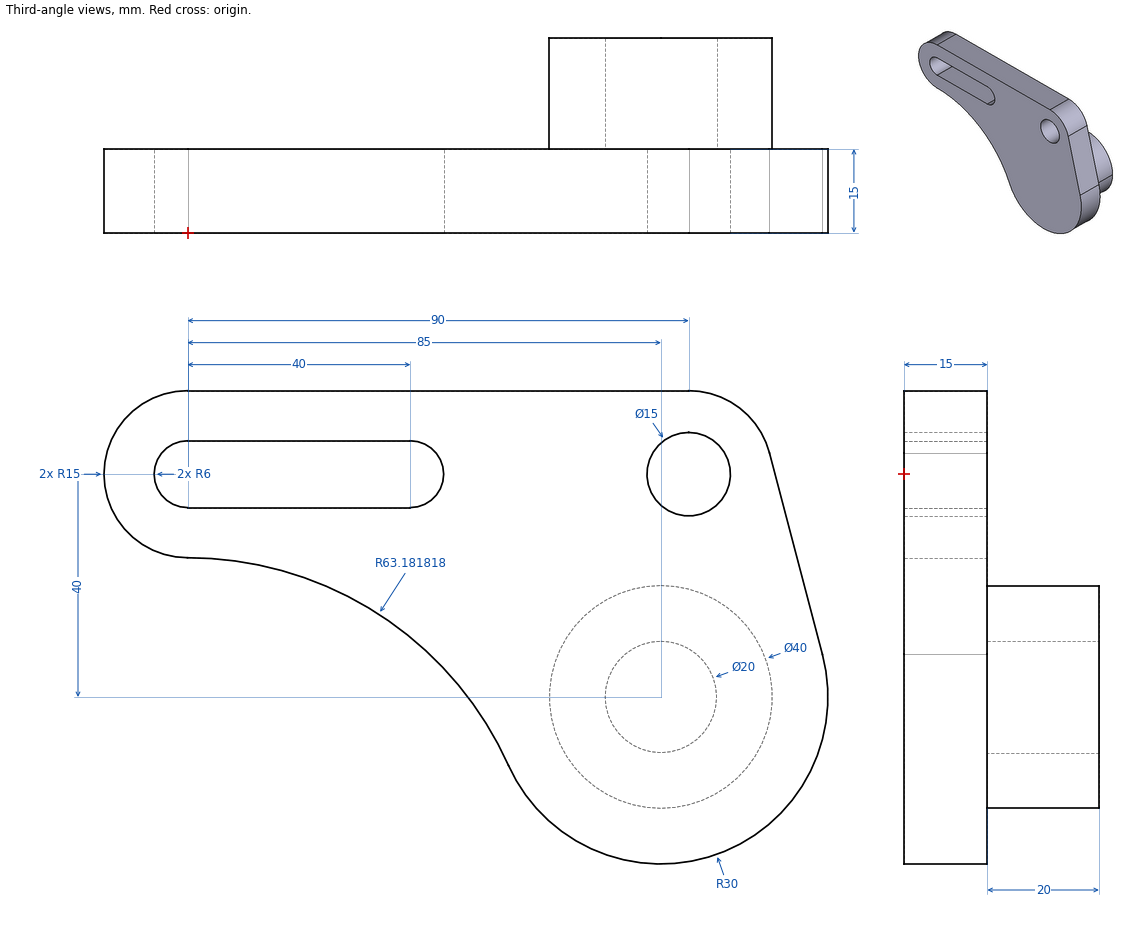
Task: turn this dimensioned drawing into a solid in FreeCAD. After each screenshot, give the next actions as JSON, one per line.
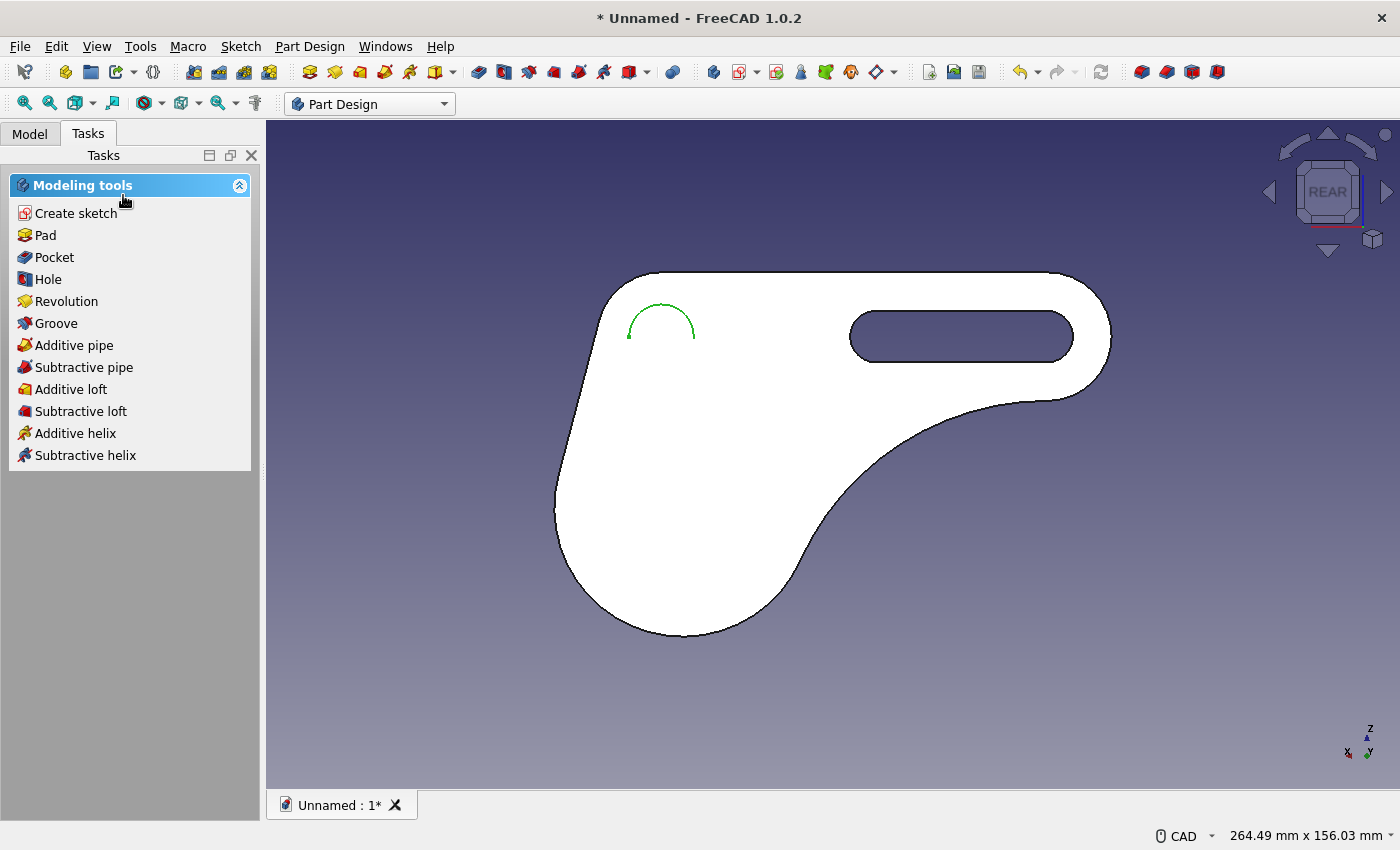
{"action": "left_click", "coordinate": [479, 72]}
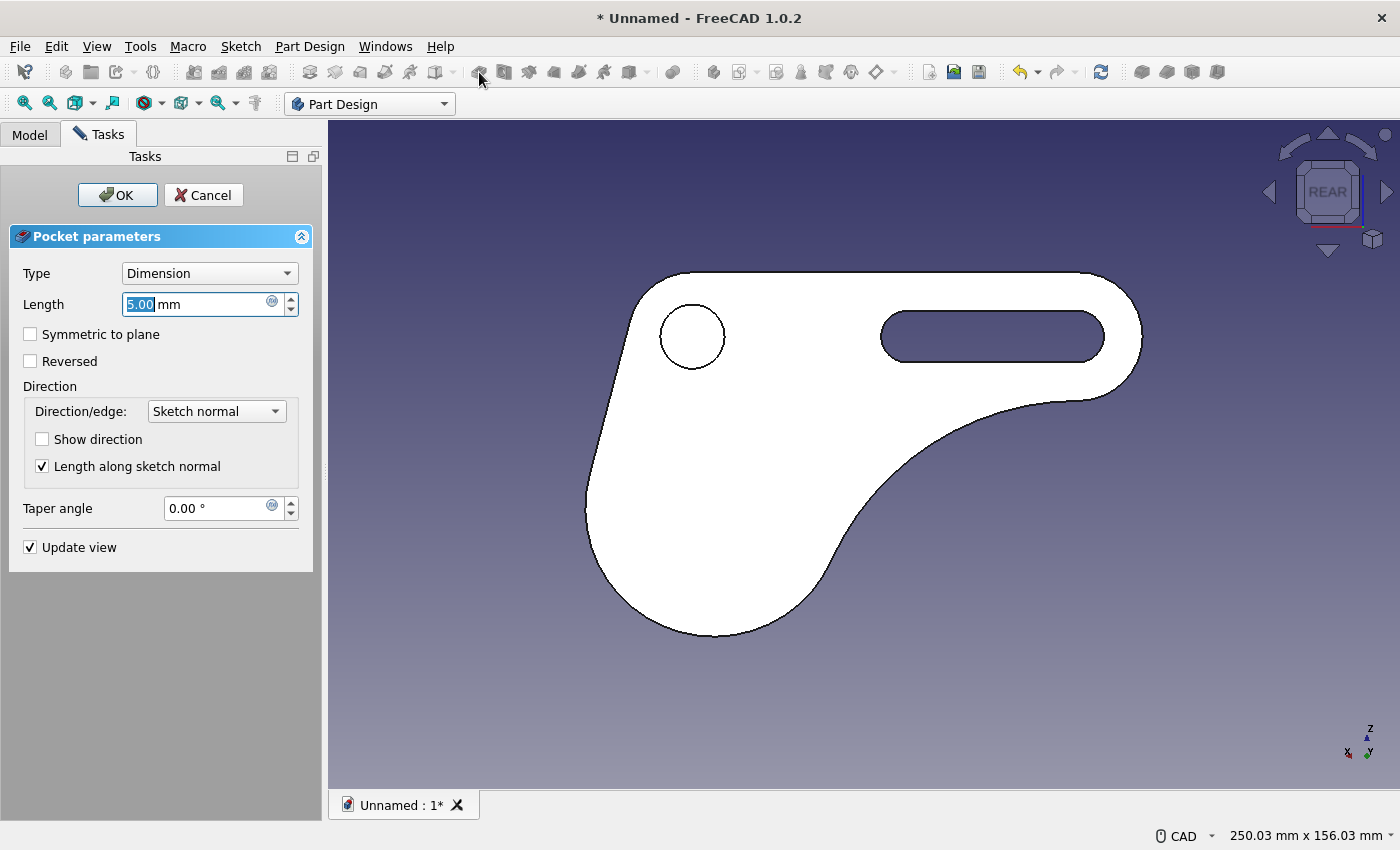
{"action": "type", "text": "15"}
{"action": "key", "text": "Tab"}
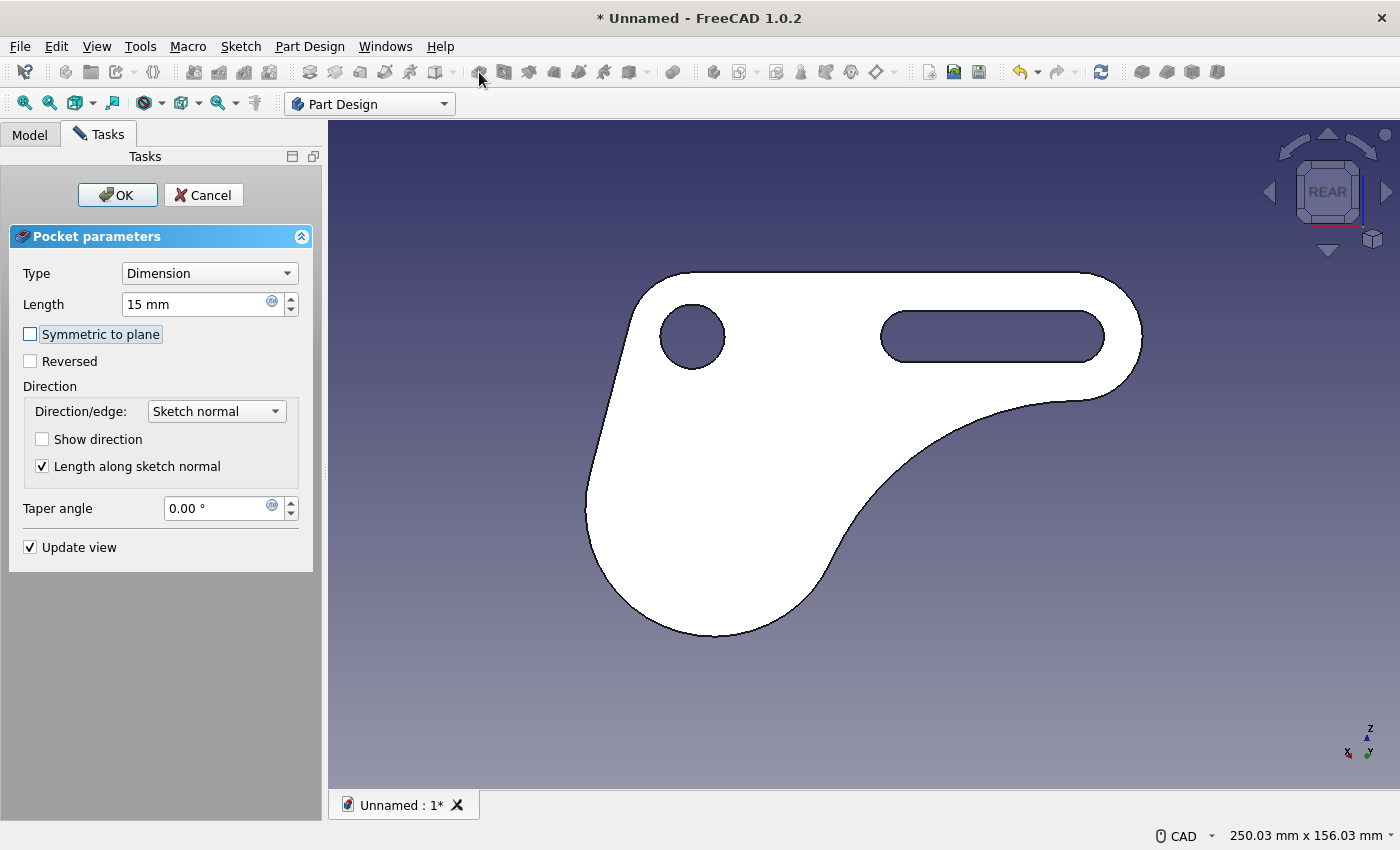
{"action": "left_click", "coordinate": [118, 195]}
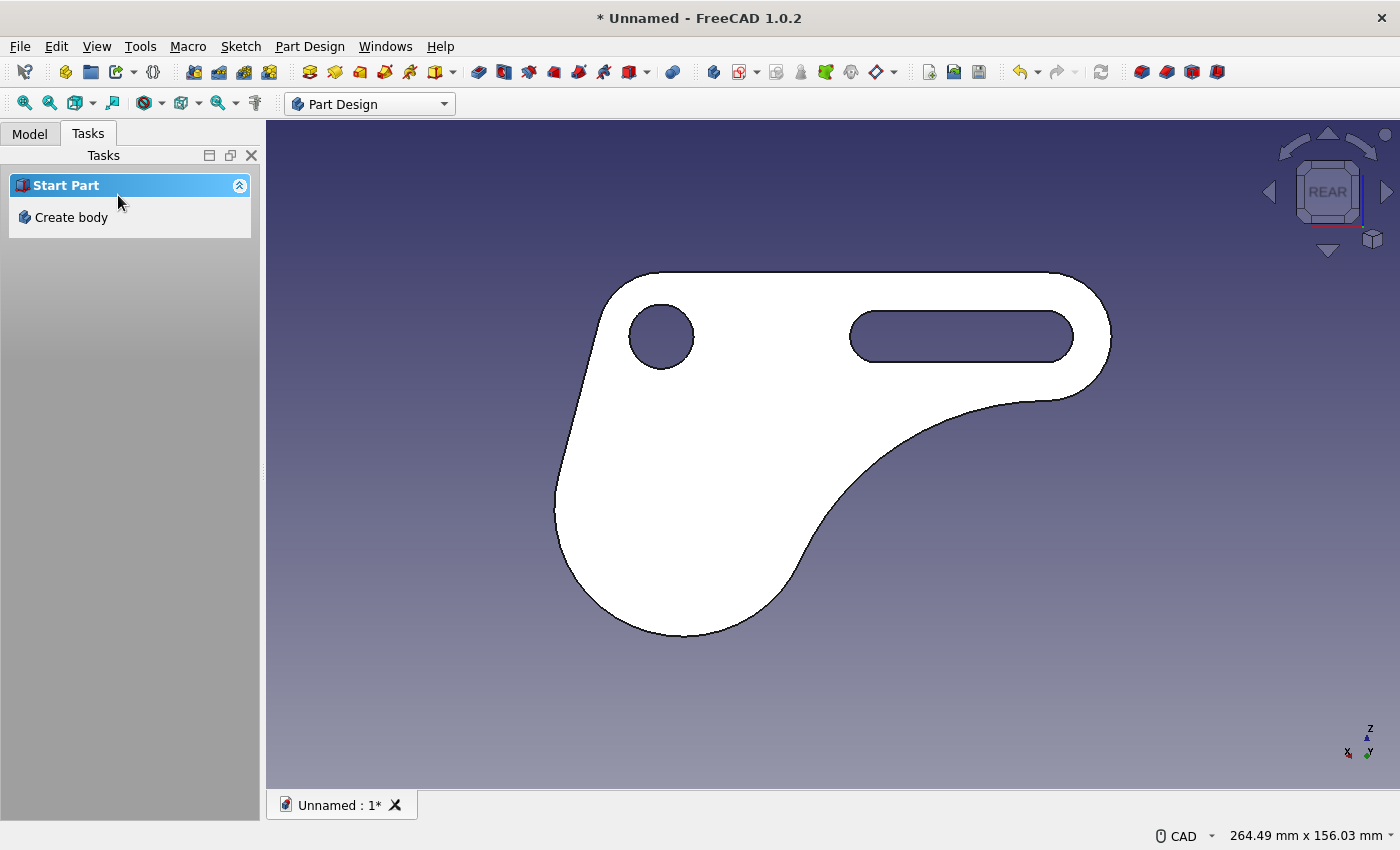
{"action": "left_click", "coordinate": [674, 506]}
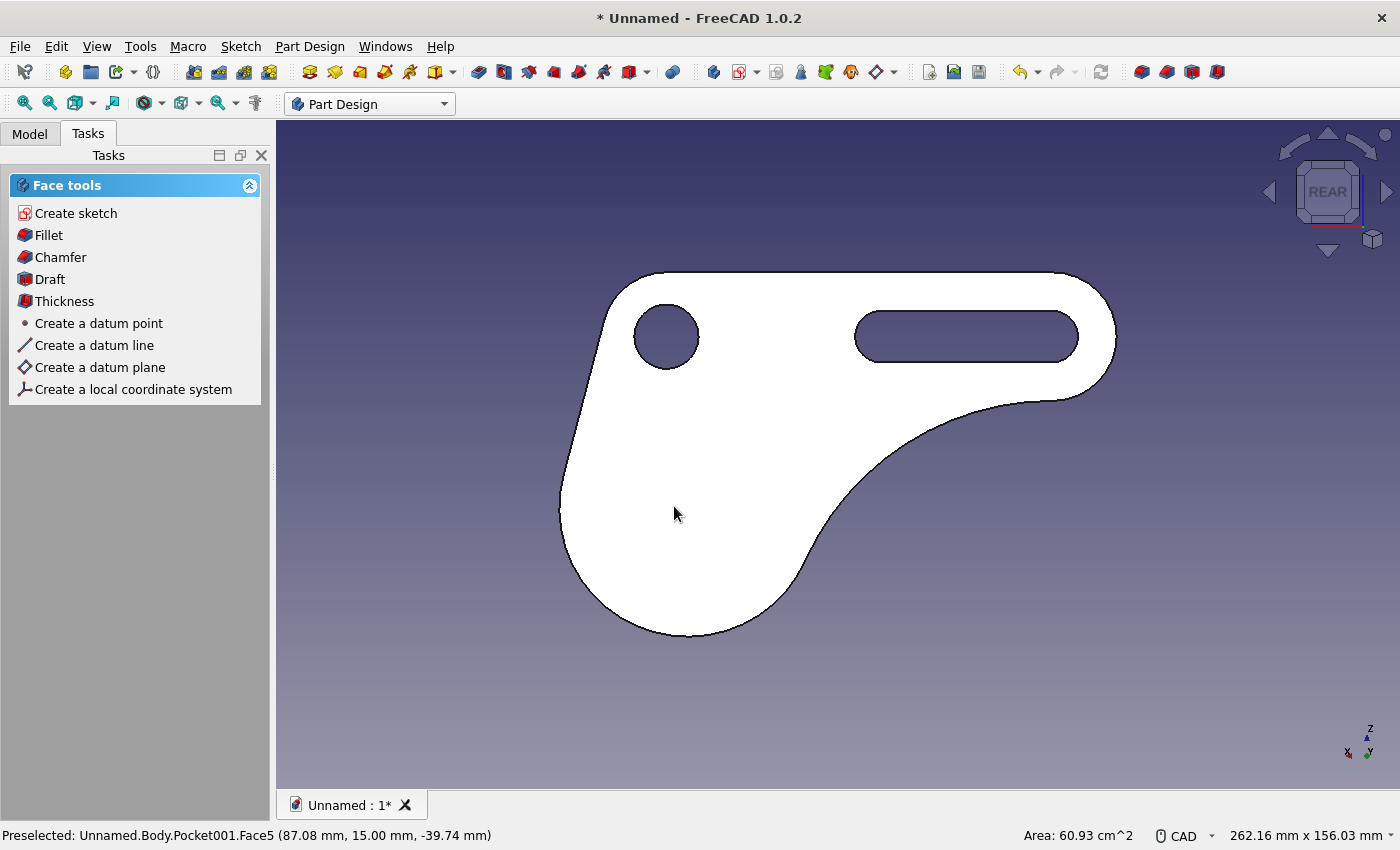
{"action": "left_click", "coordinate": [738, 72]}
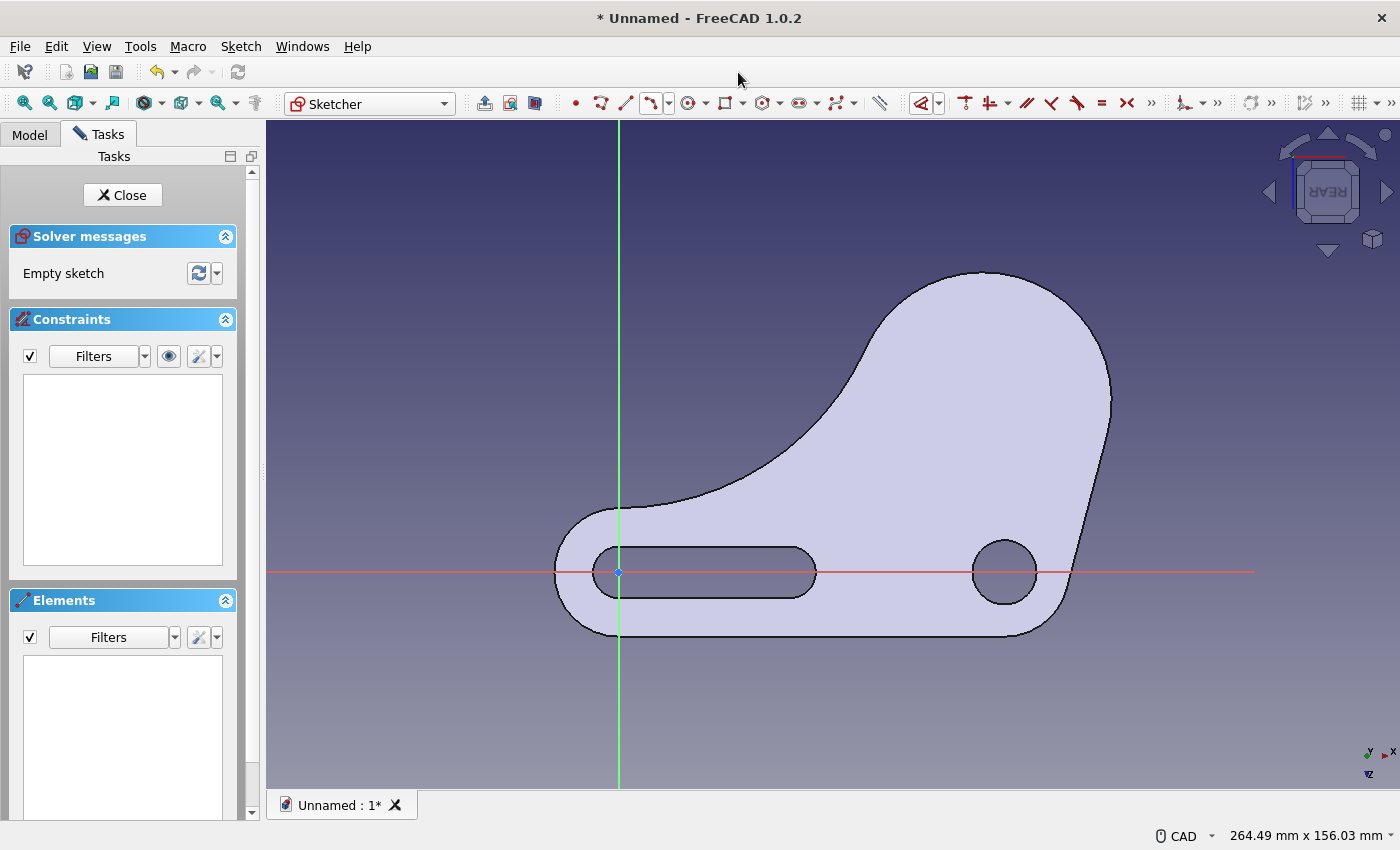
{"action": "scroll", "coordinate": [1110, 370], "scroll_direction": "up", "scroll_amount": 5}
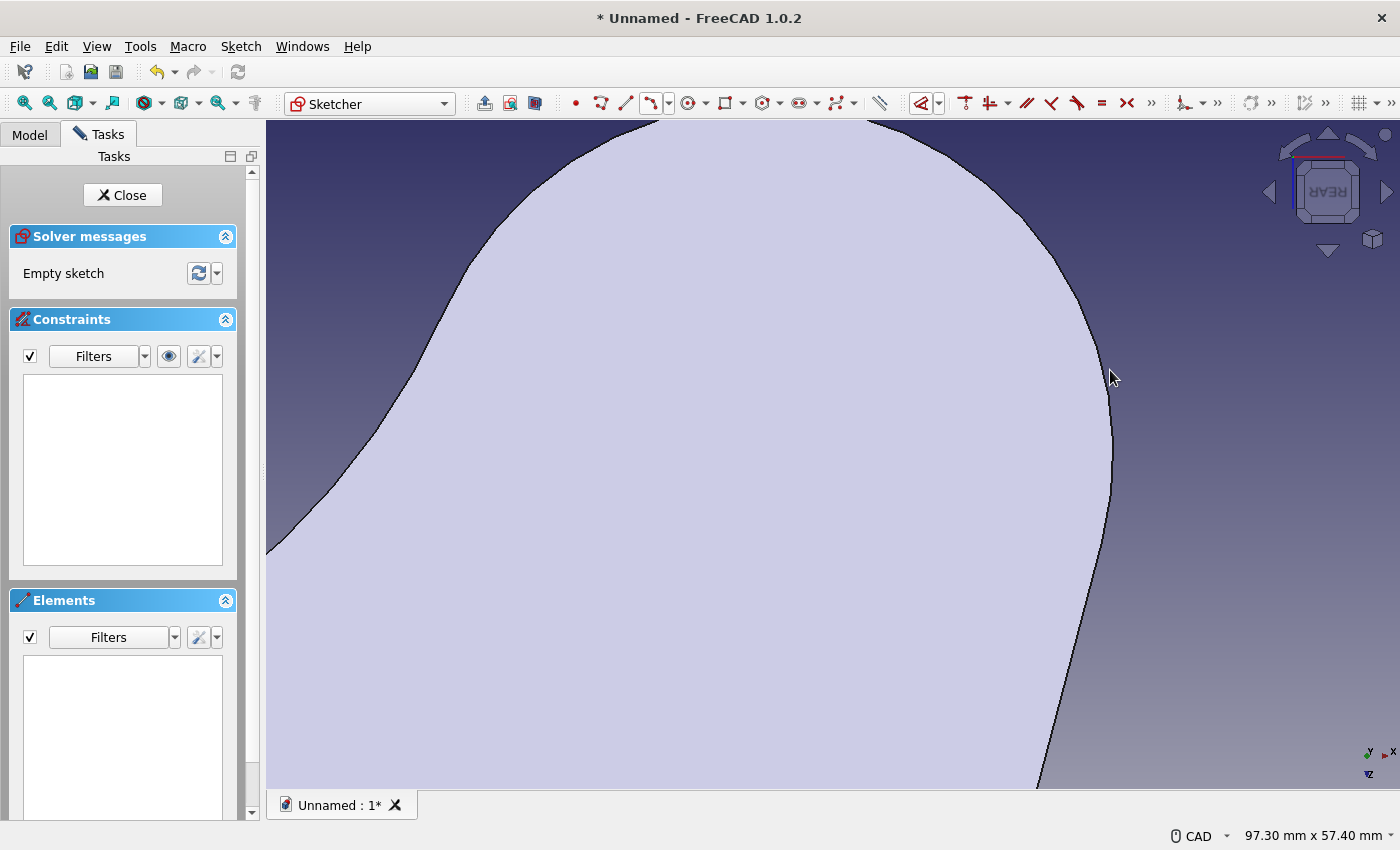
{"action": "left_click", "coordinate": [688, 104]}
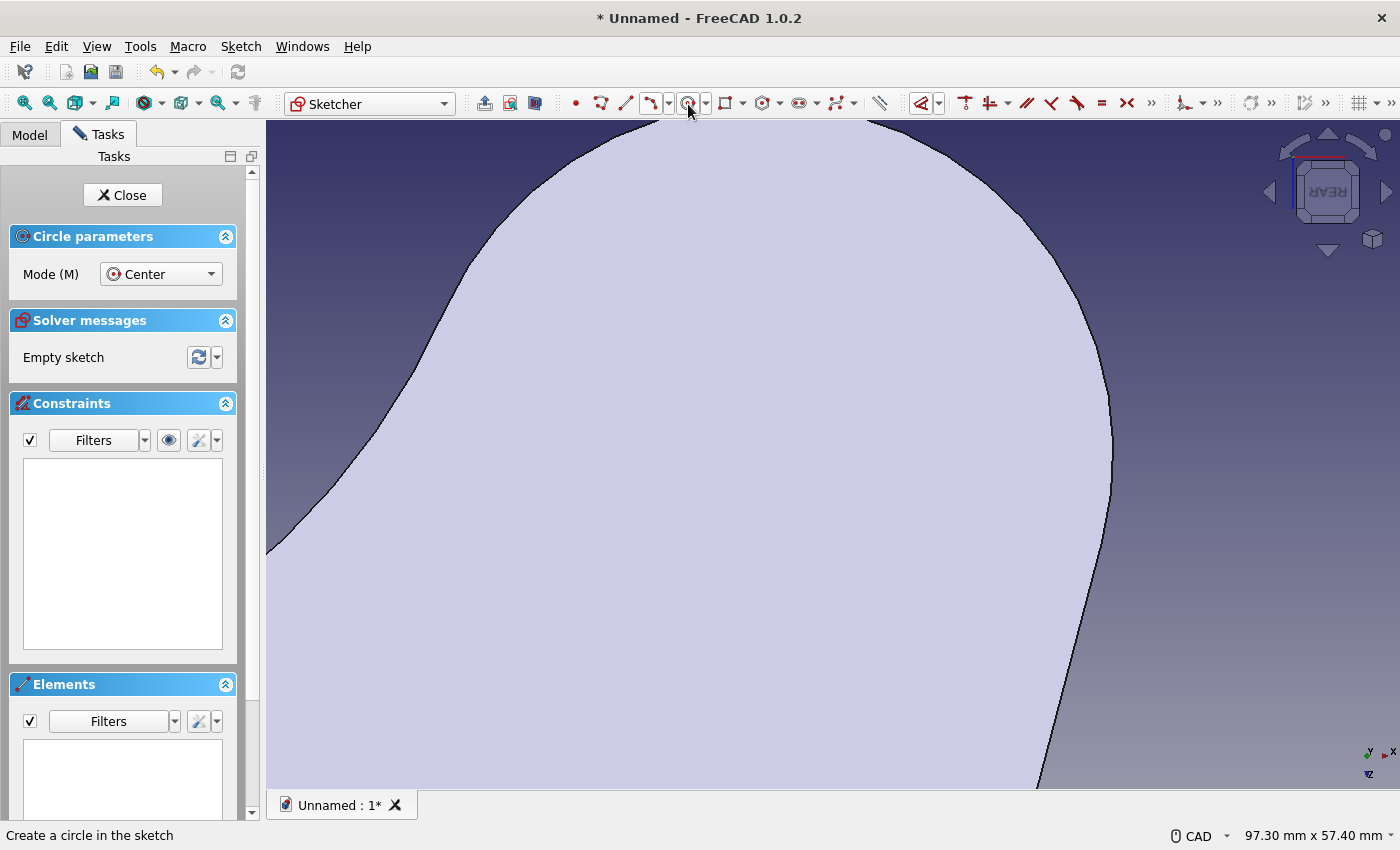
{"action": "left_click", "coordinate": [764, 453]}
{"action": "left_click", "coordinate": [929, 289]}